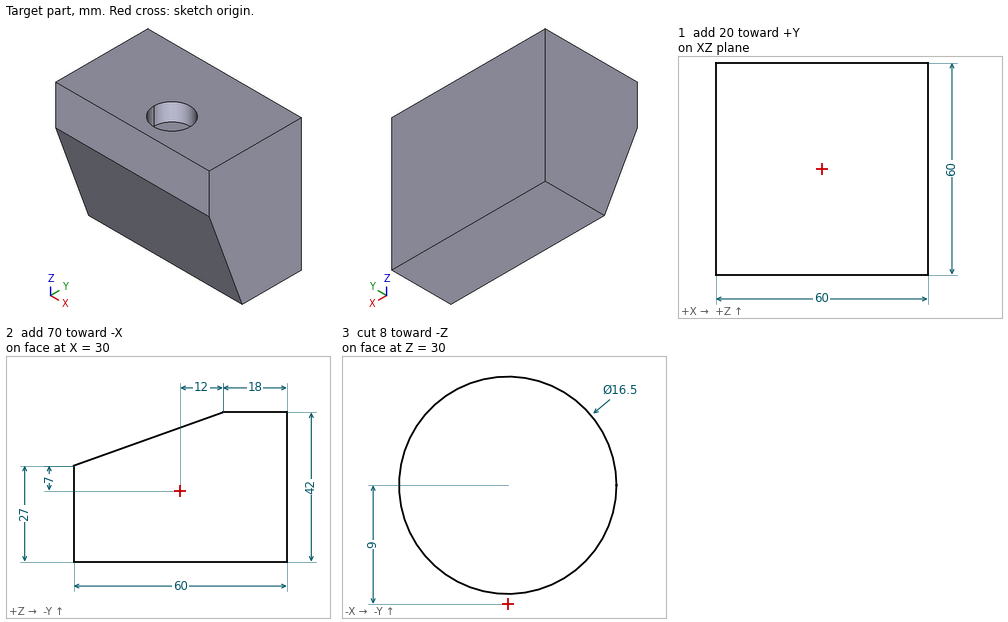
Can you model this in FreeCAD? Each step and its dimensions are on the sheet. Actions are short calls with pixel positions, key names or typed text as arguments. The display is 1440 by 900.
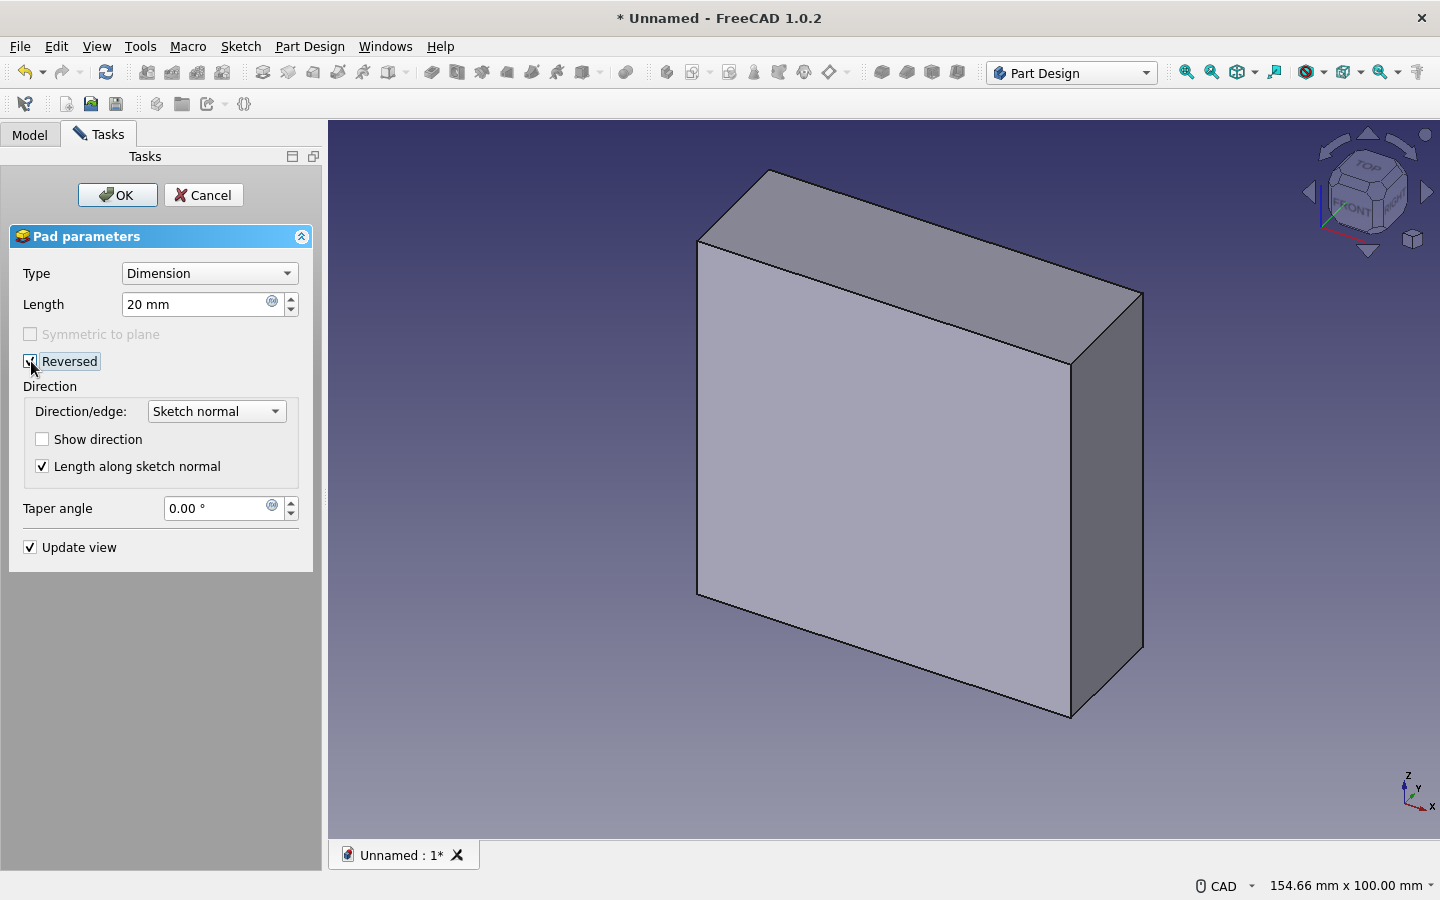
click(118, 195)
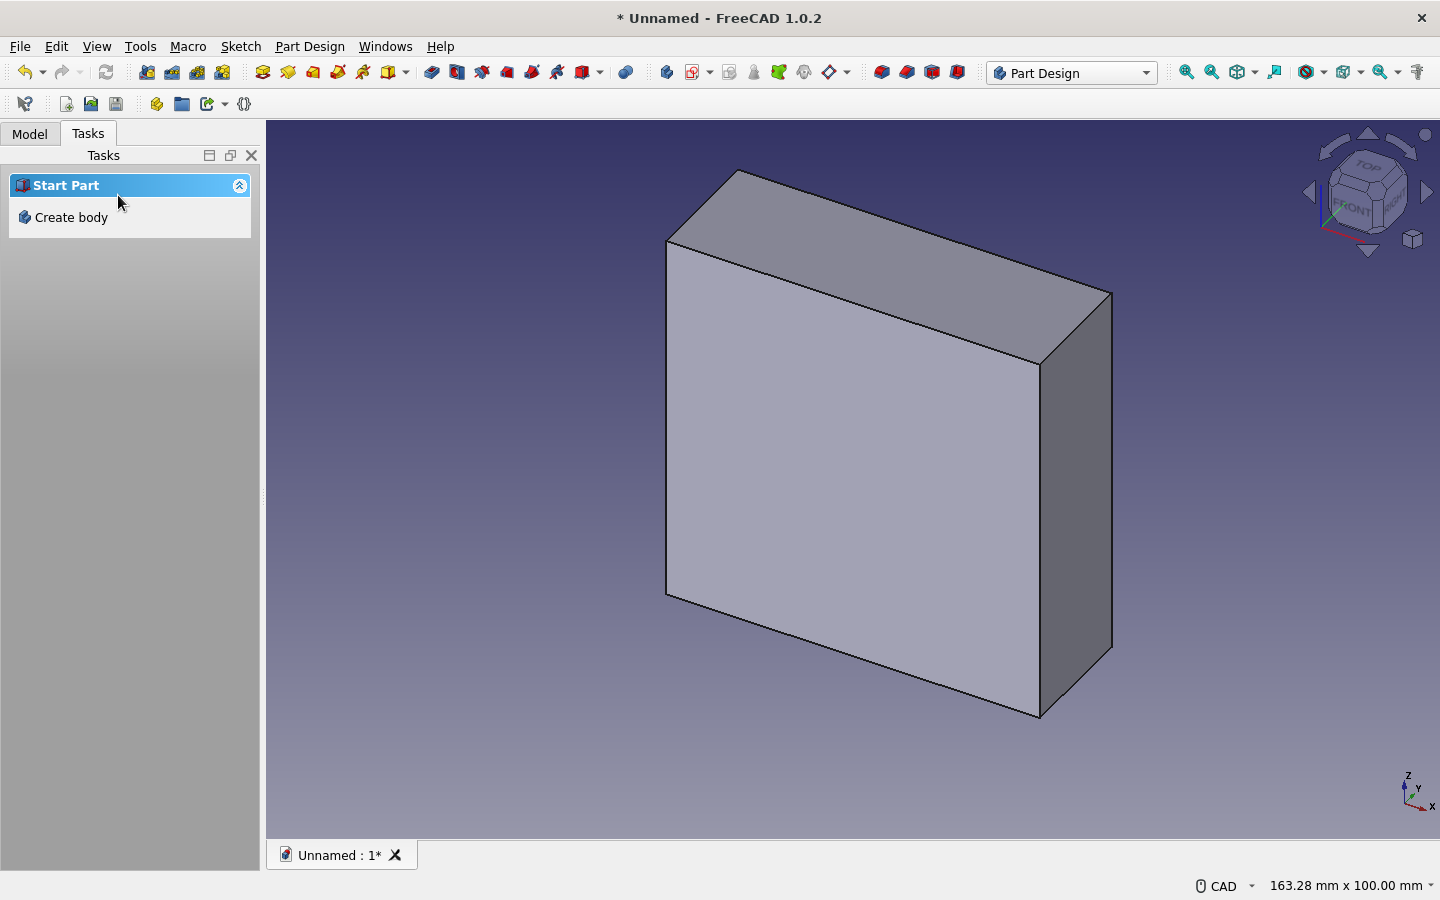
click(1076, 404)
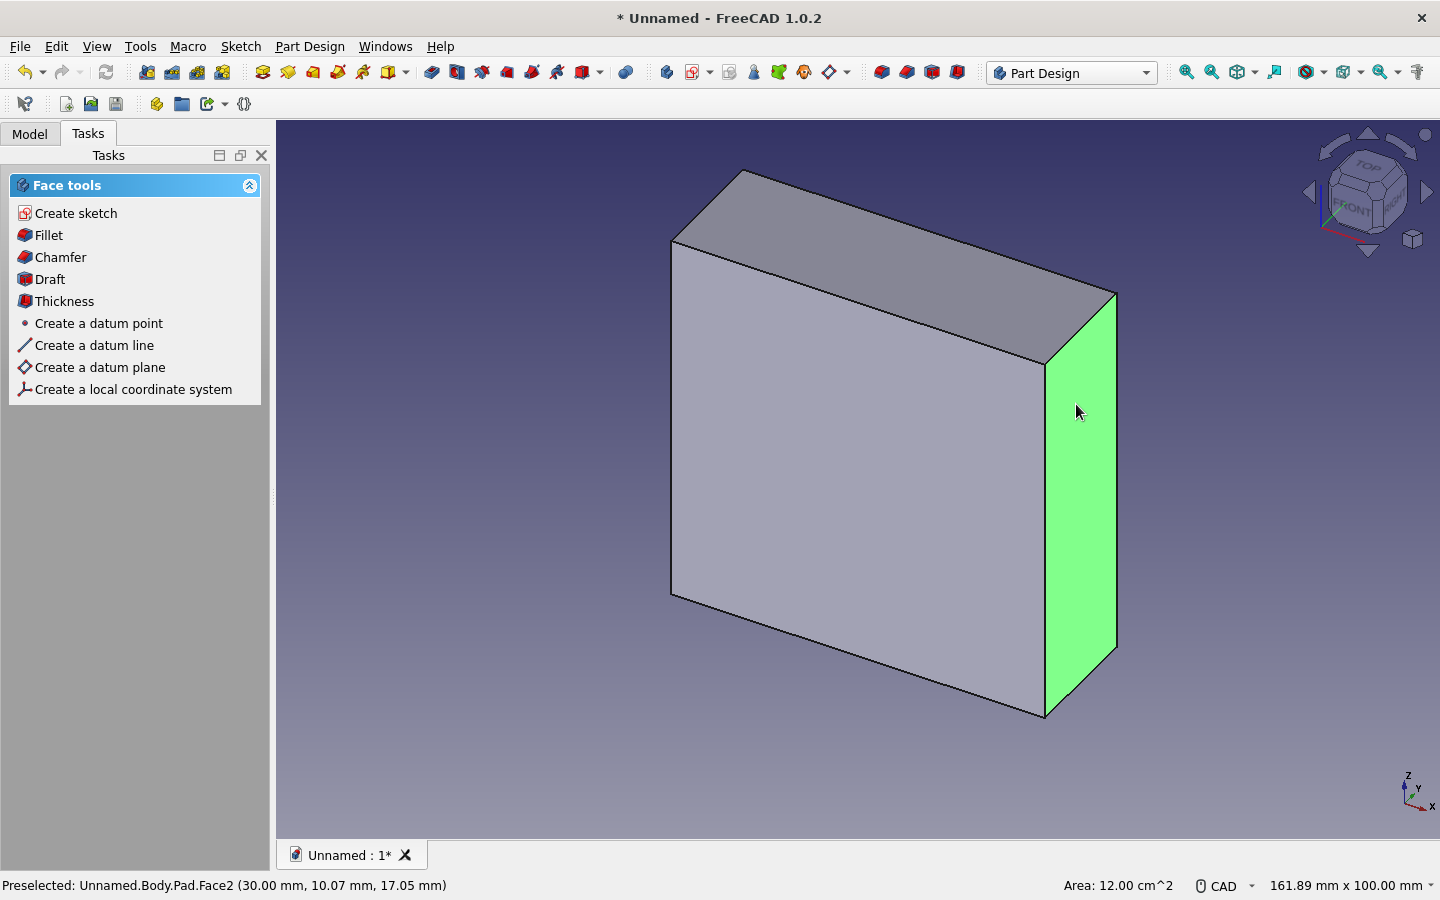
click(692, 72)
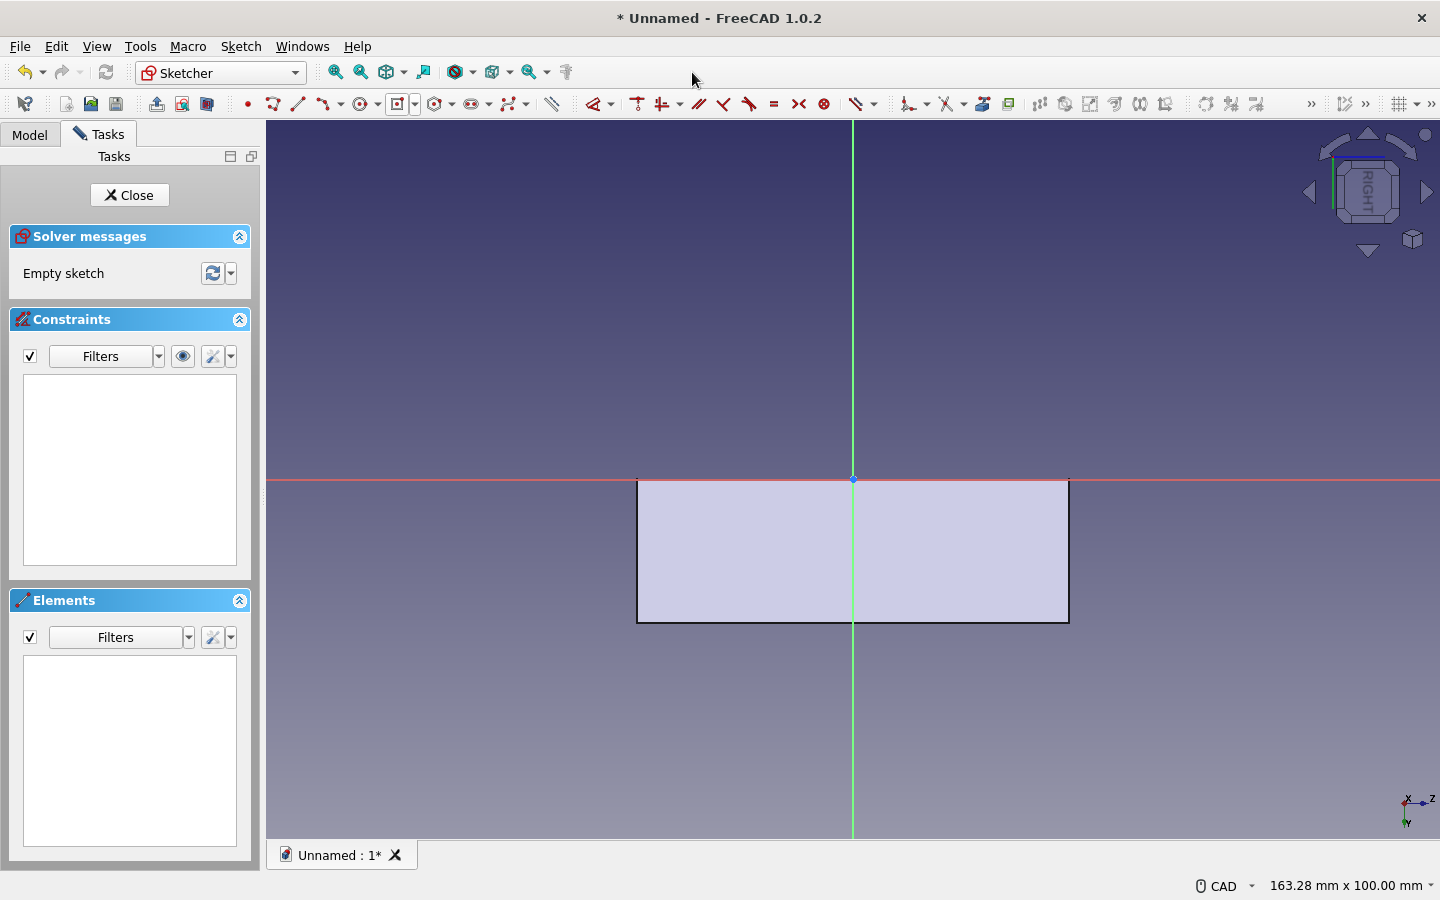
scroll(992, 458, up, 2)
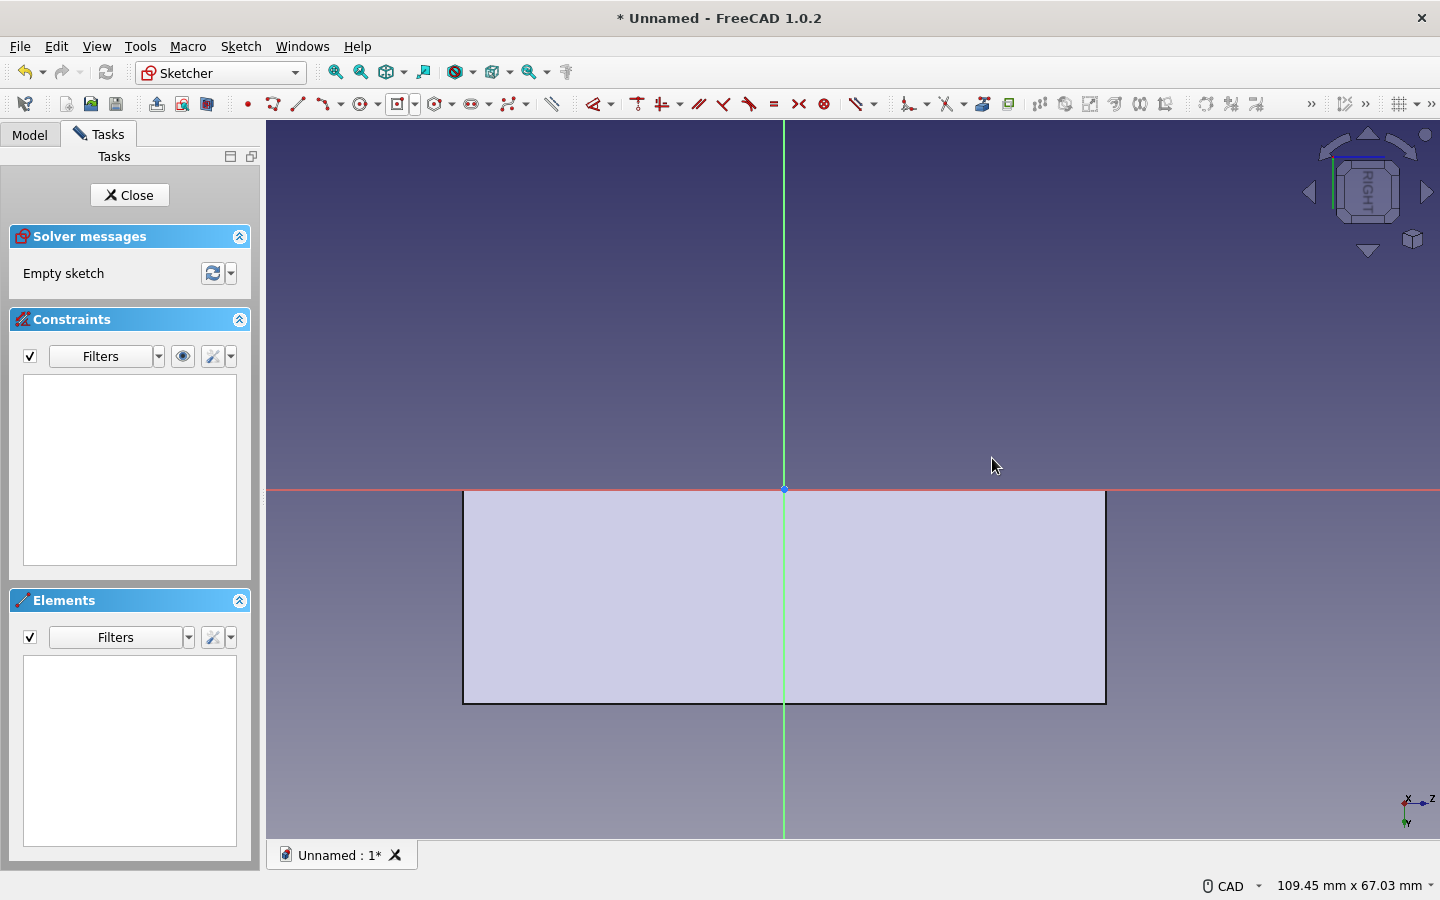
click(273, 104)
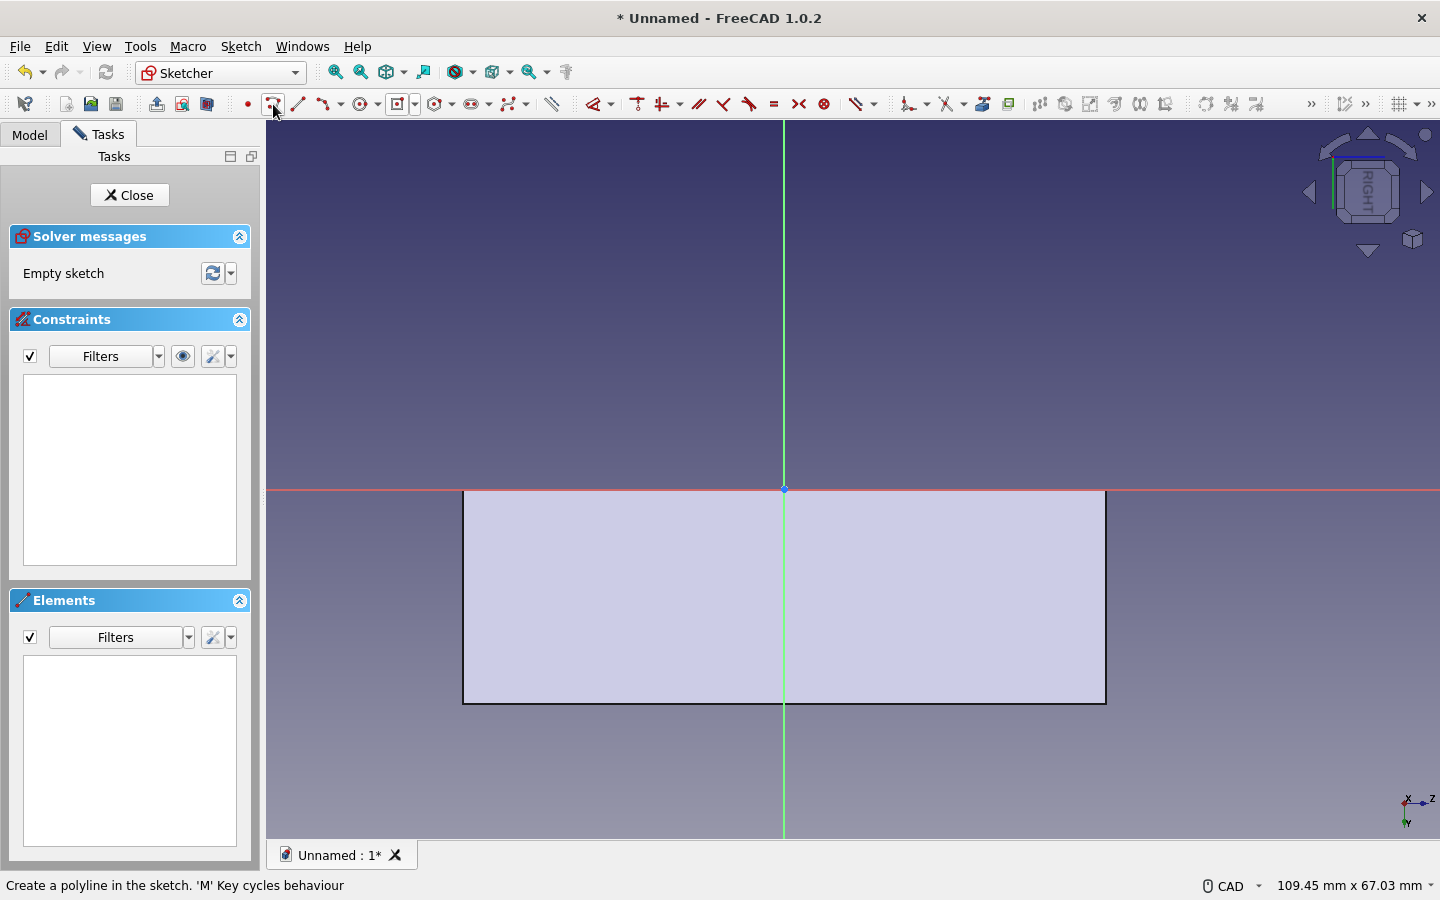
click(913, 254)
click(463, 415)
click(463, 704)
click(1106, 704)
click(1106, 254)
click(913, 255)
key(Escape)
key(Escape)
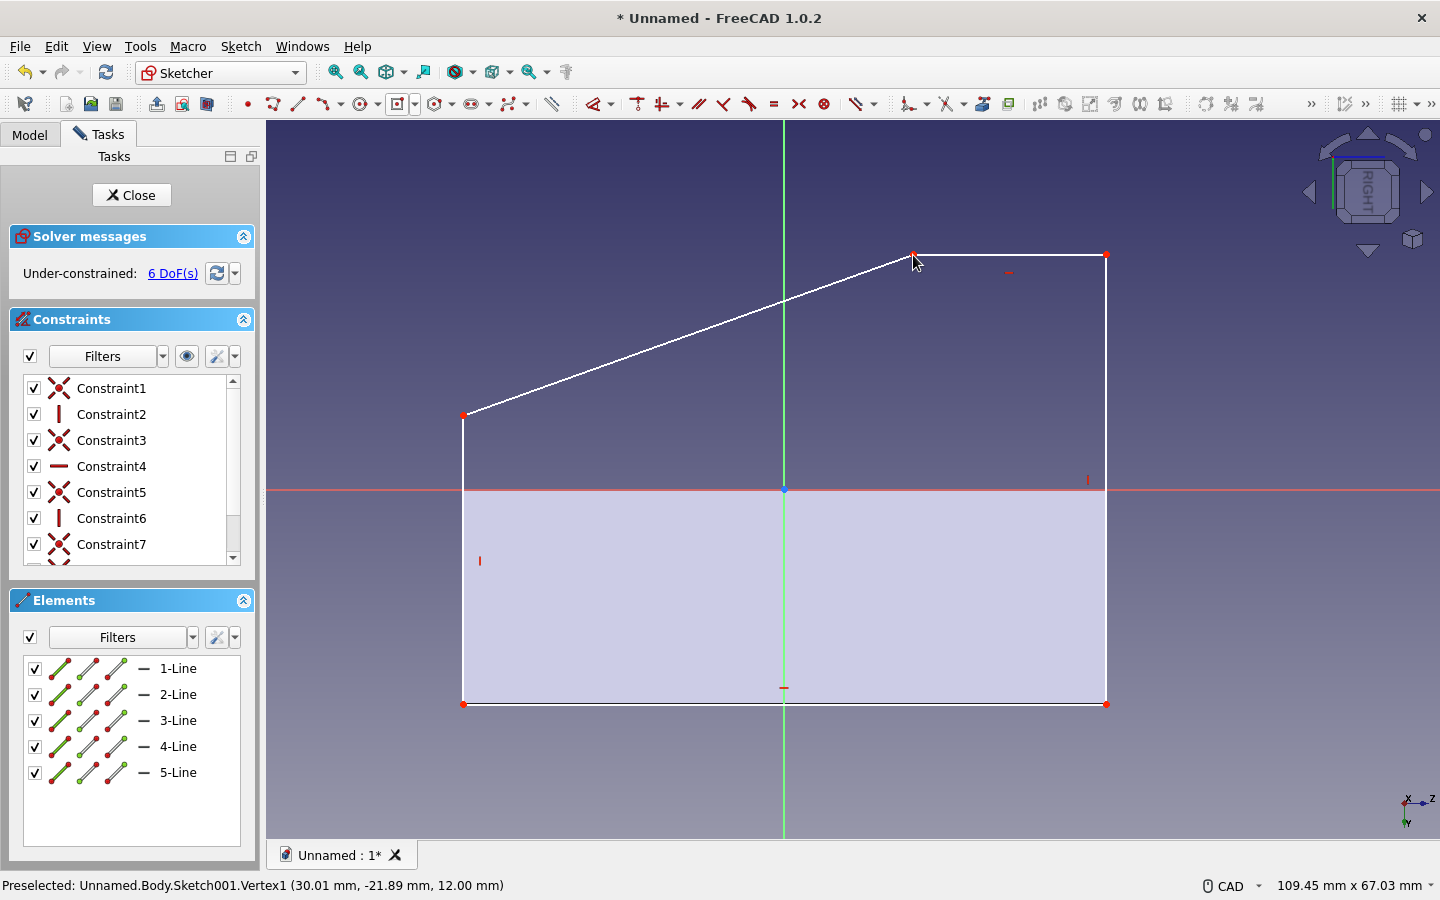
key(d)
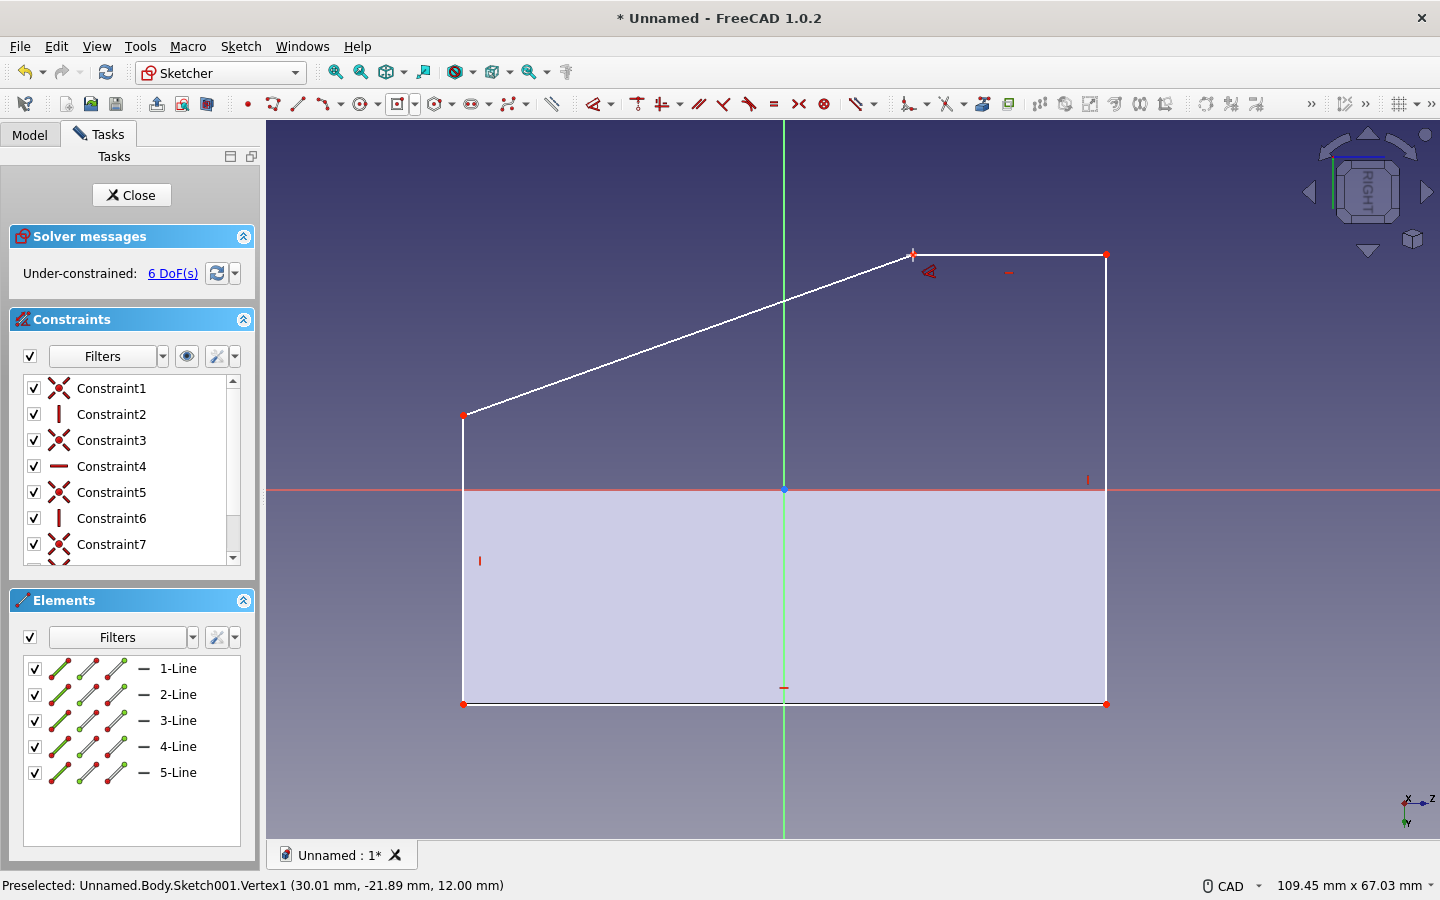
click(463, 503)
click(429, 561)